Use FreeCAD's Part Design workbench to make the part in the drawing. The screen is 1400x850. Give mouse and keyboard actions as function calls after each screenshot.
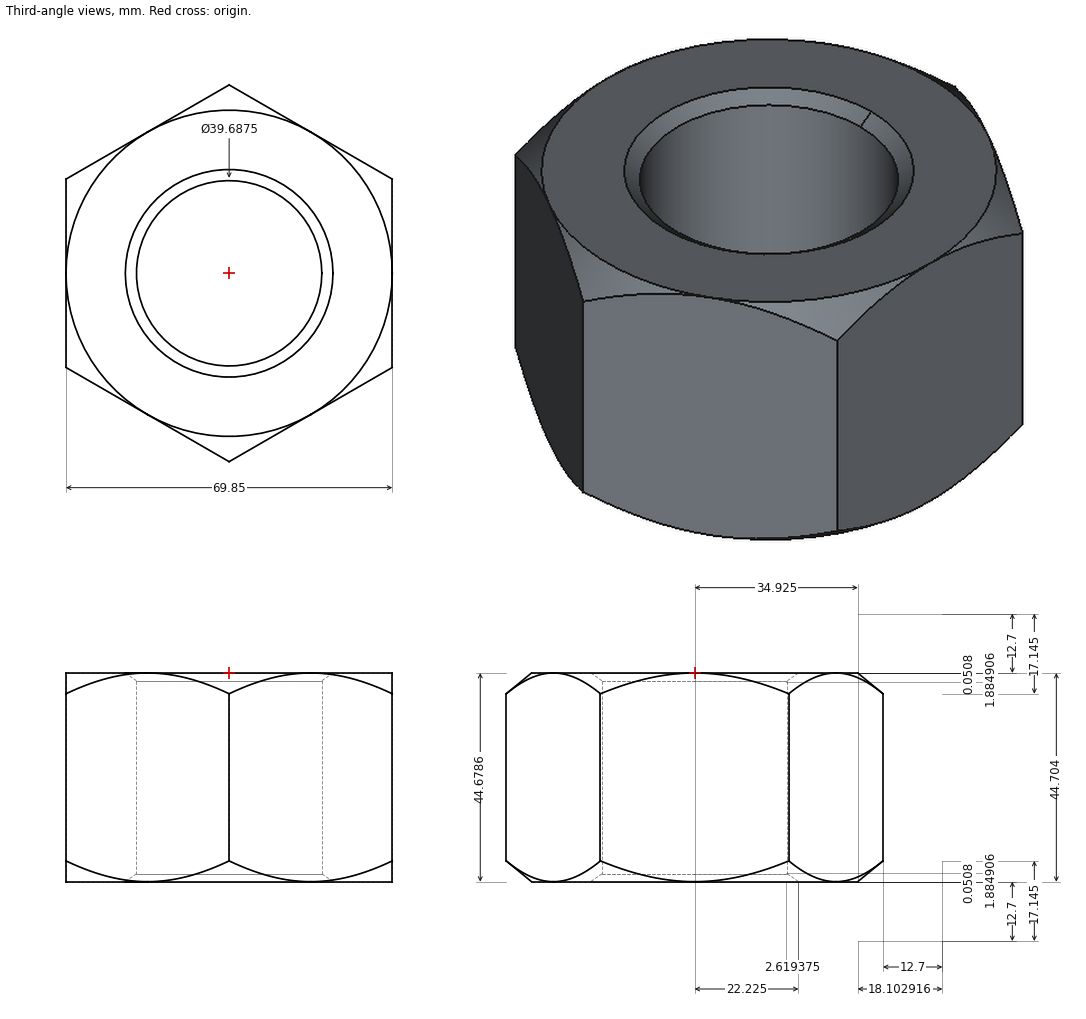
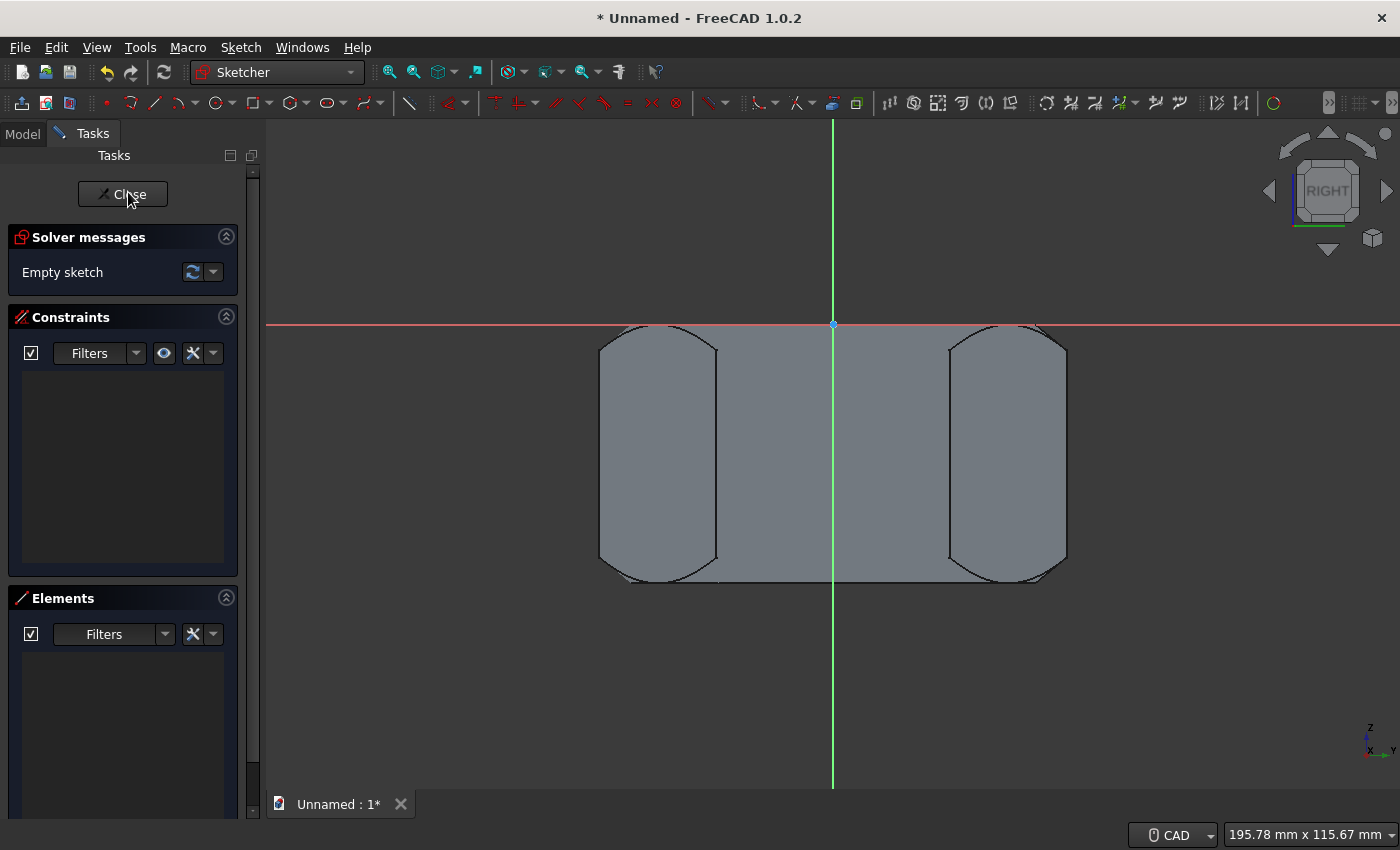
scroll(1059, 454, up, 3)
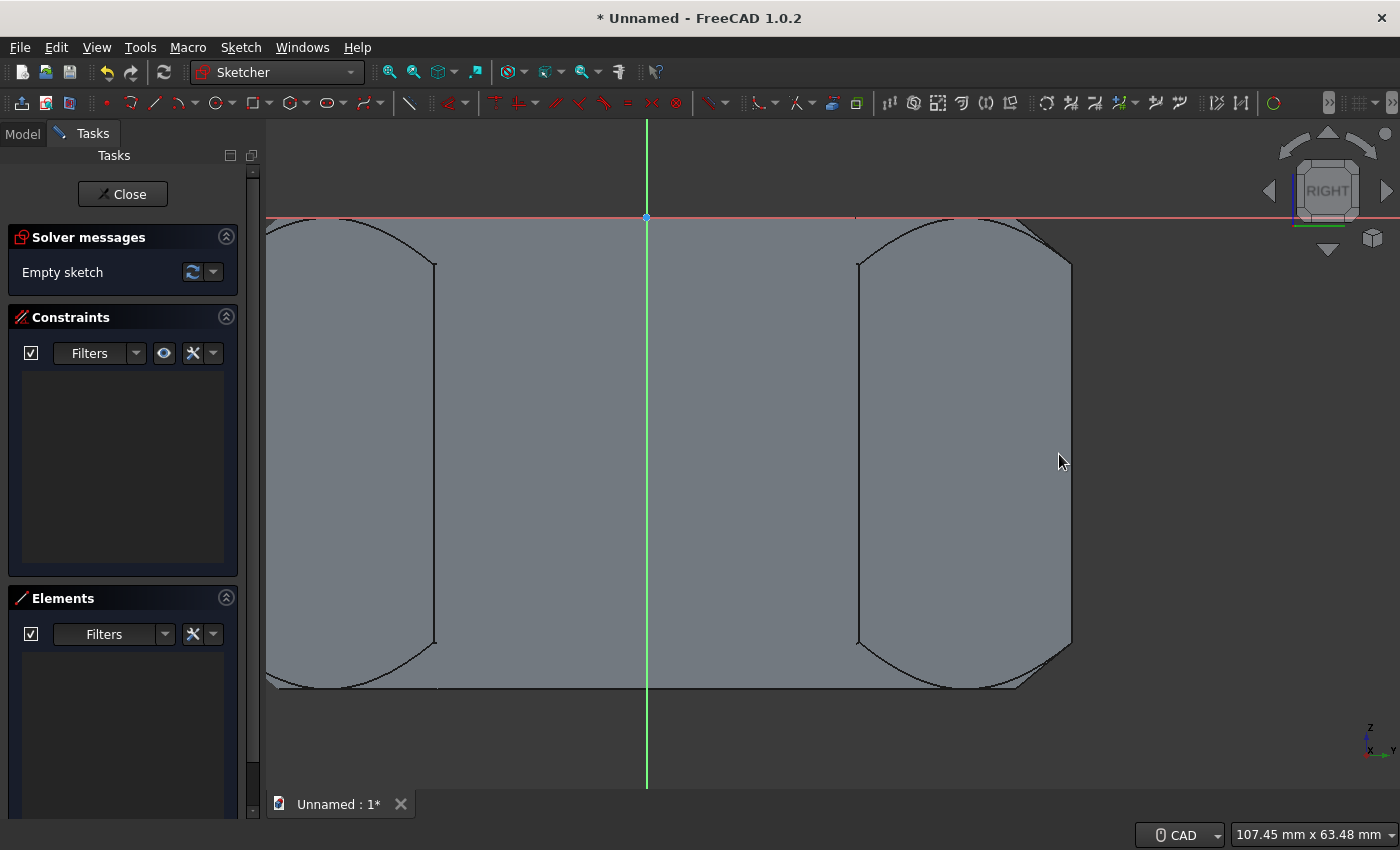
click(132, 104)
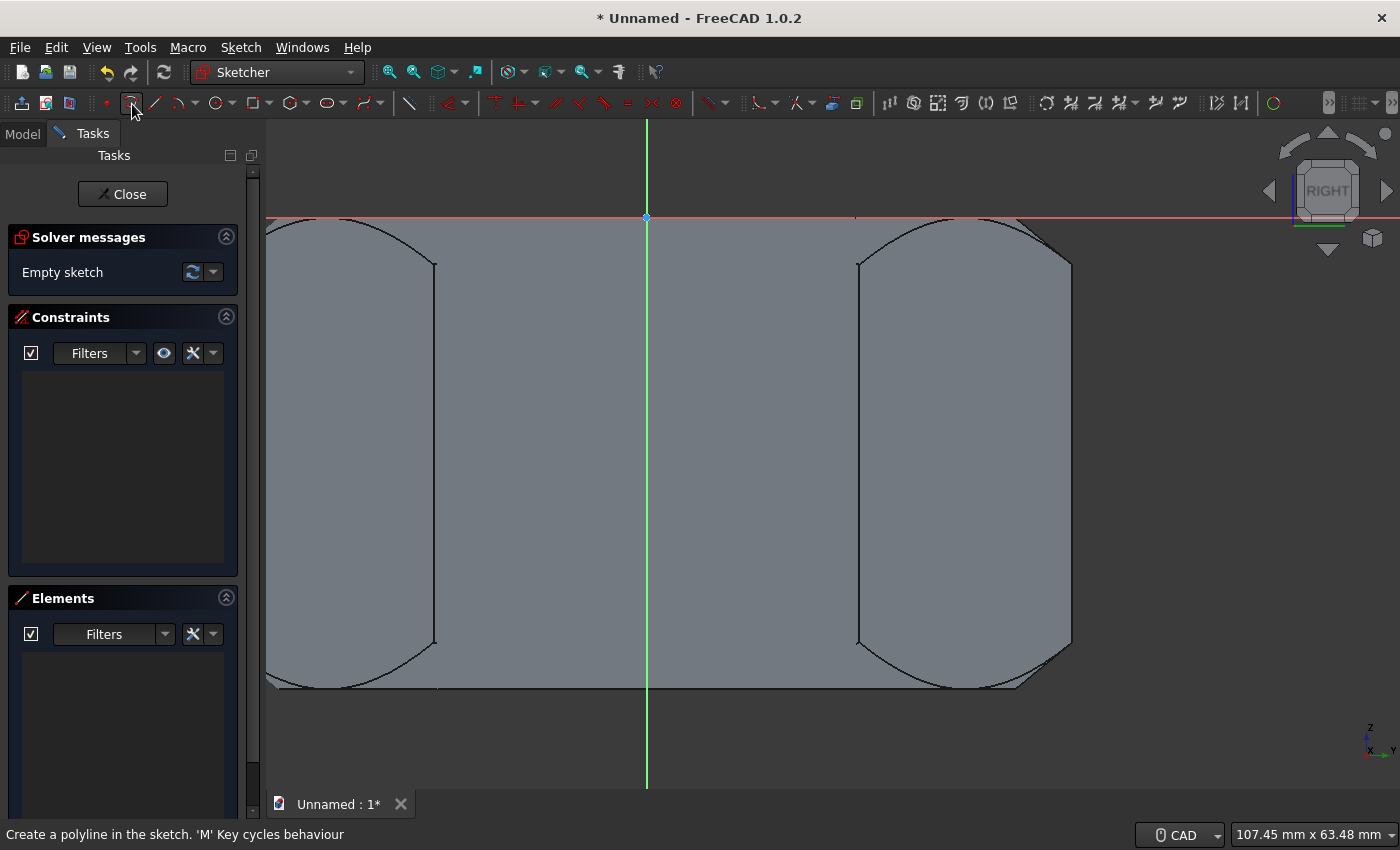
click(854, 670)
click(854, 690)
click(881, 690)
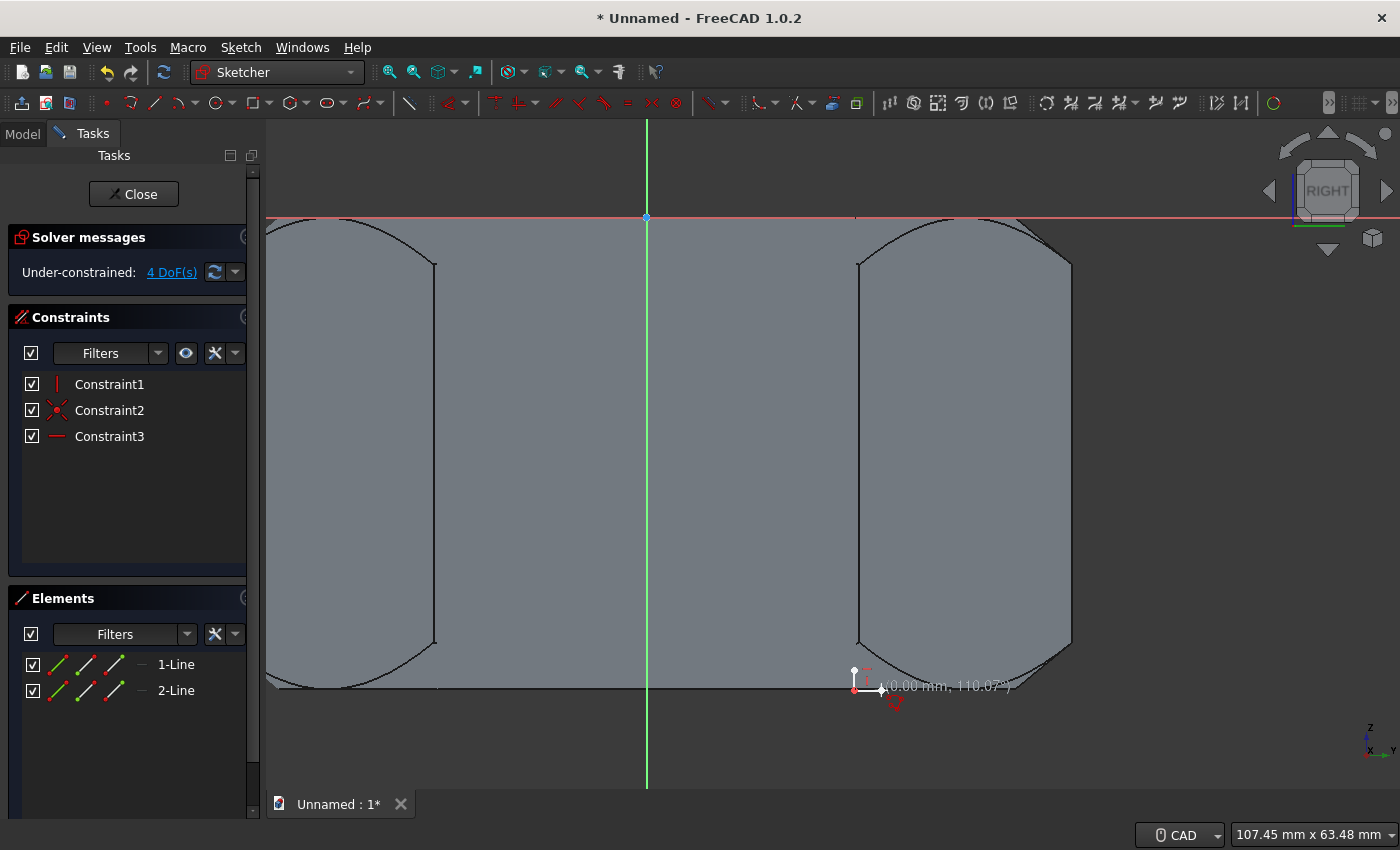
scroll(881, 689, up, 17)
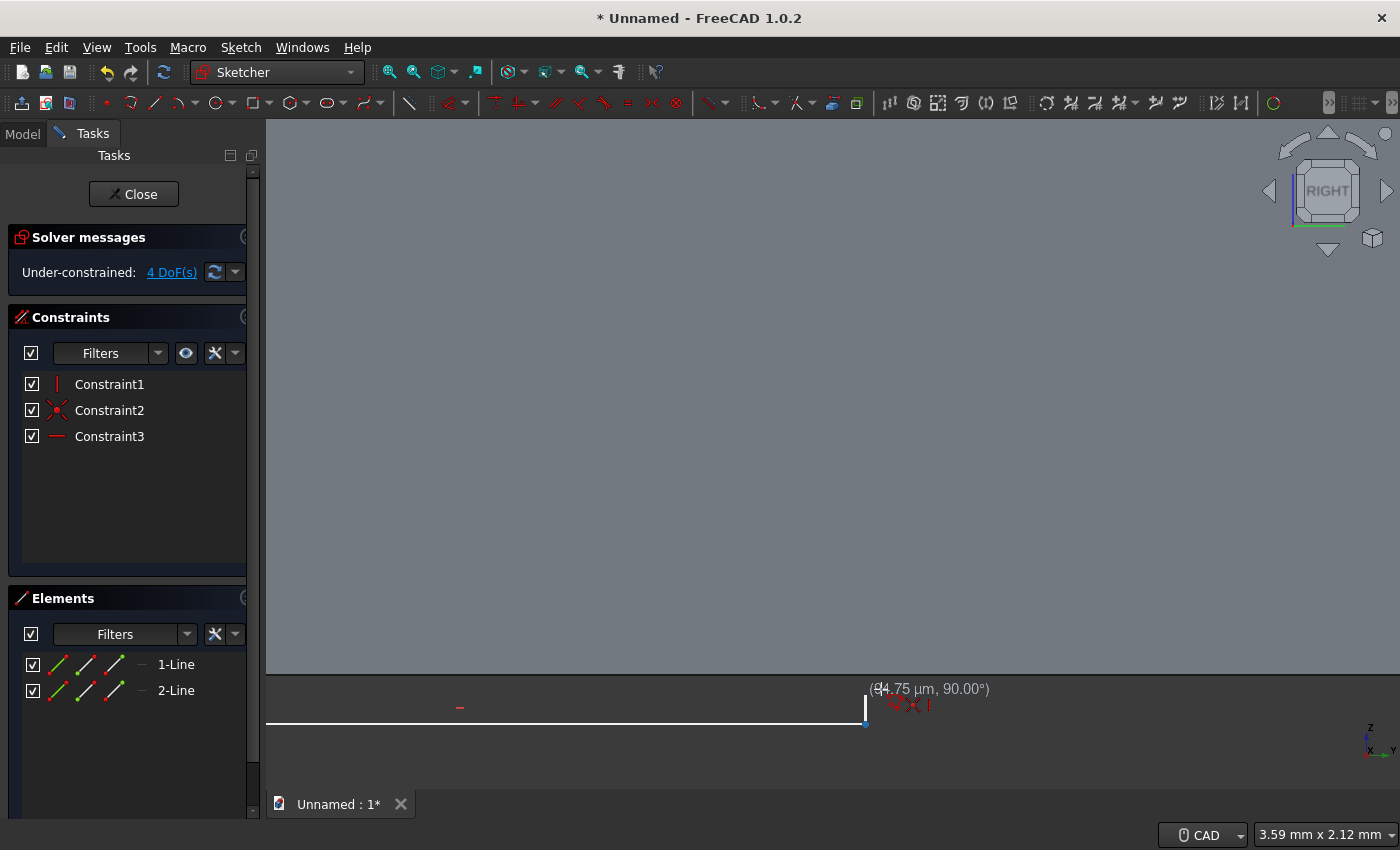
click(865, 667)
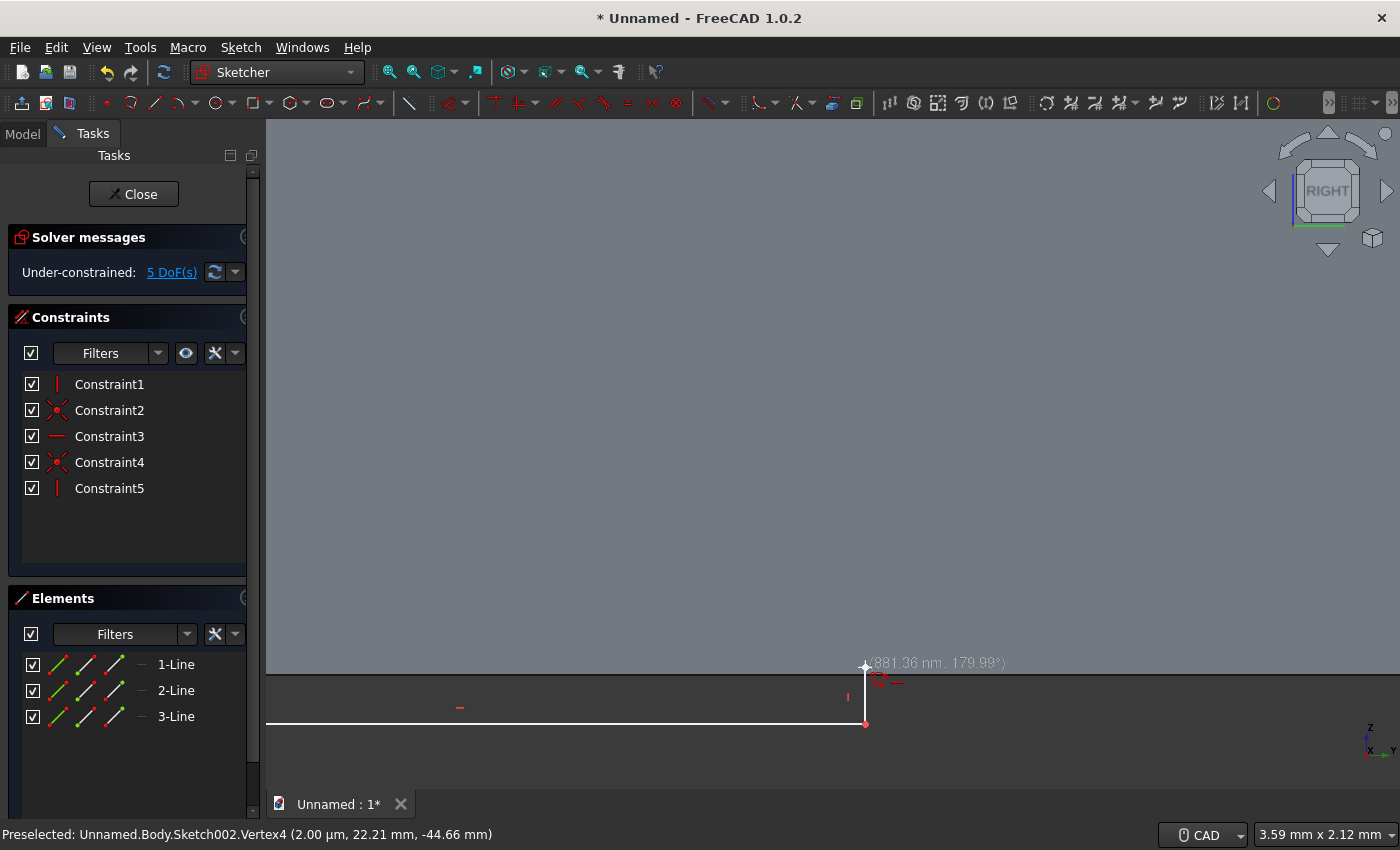
scroll(882, 690, down, 17)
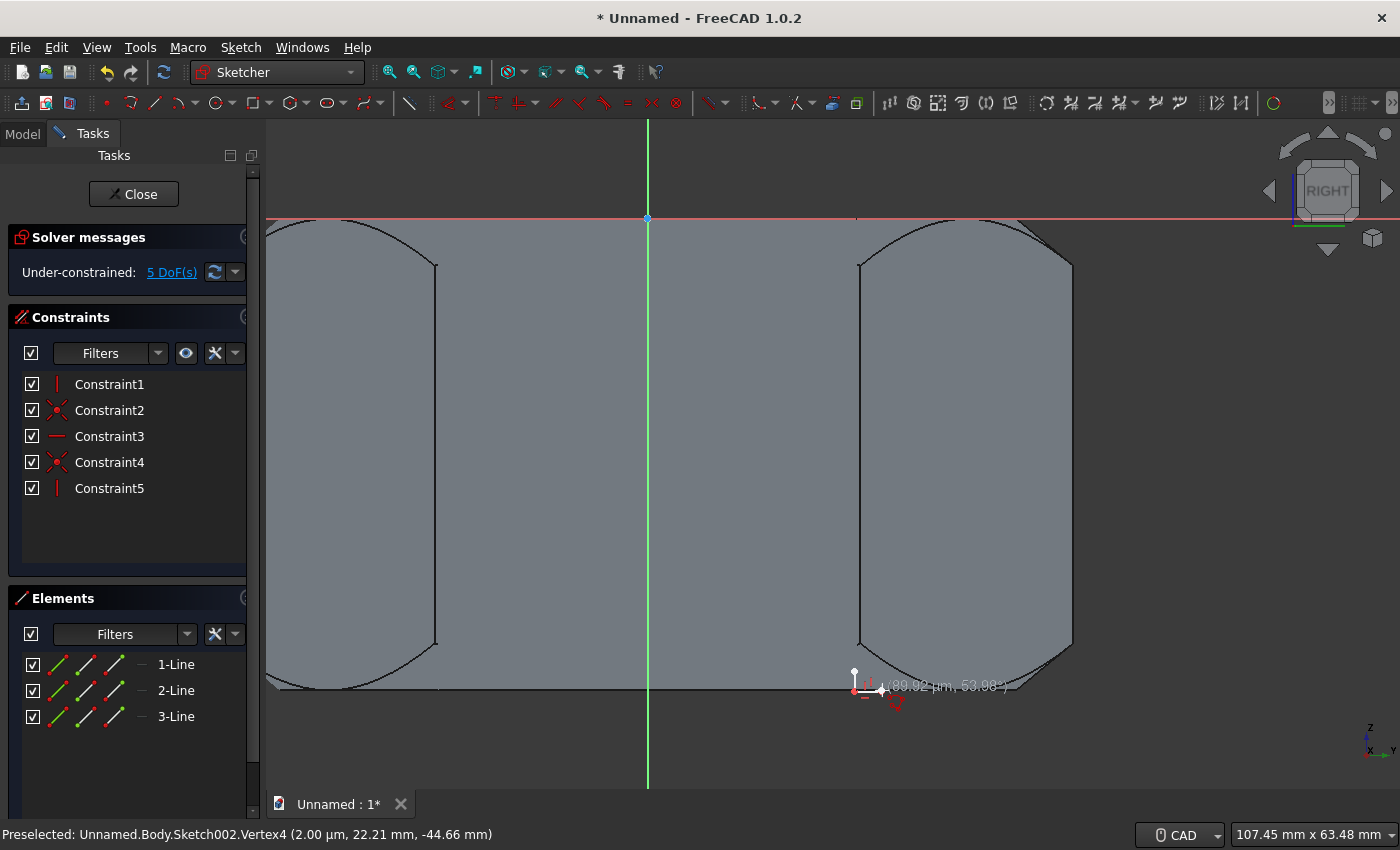
scroll(855, 671, up, 3)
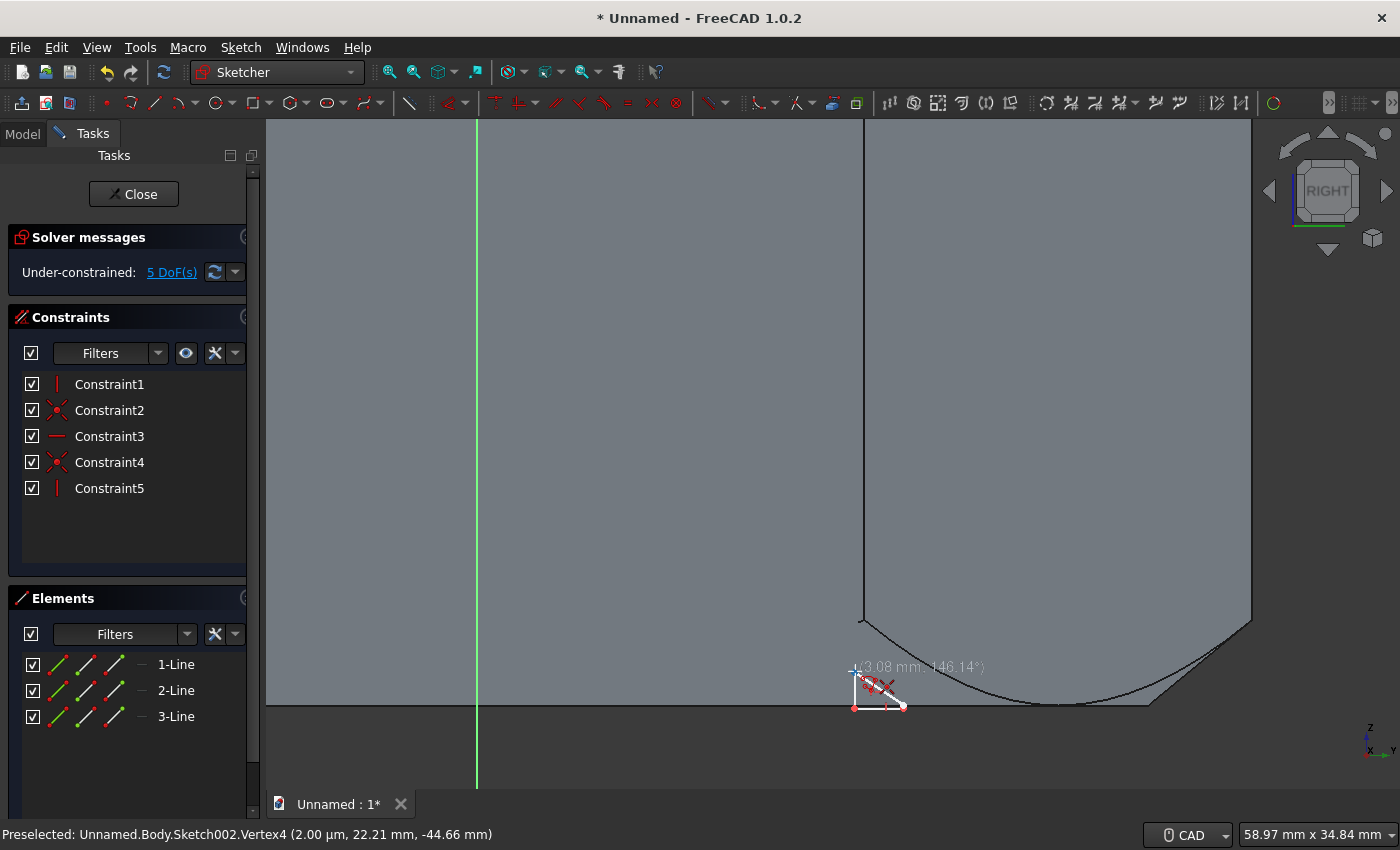
click(855, 672)